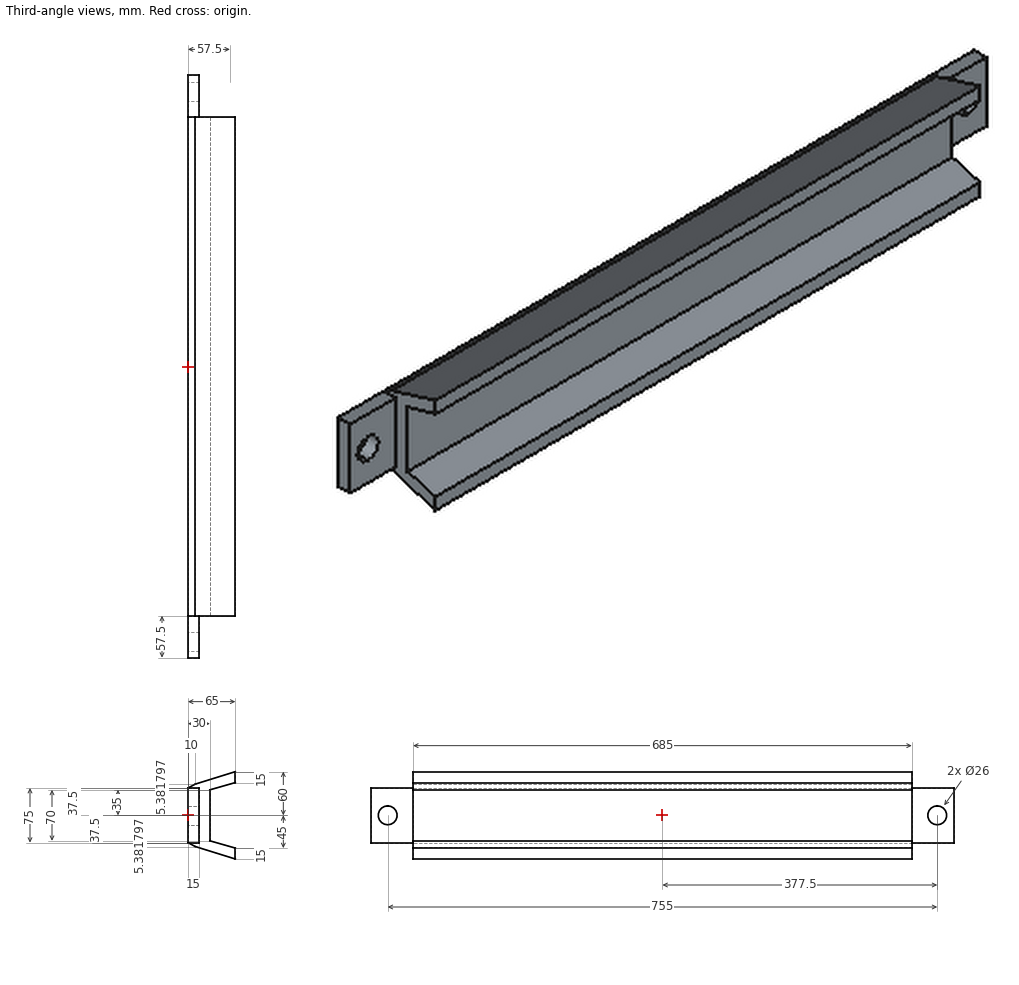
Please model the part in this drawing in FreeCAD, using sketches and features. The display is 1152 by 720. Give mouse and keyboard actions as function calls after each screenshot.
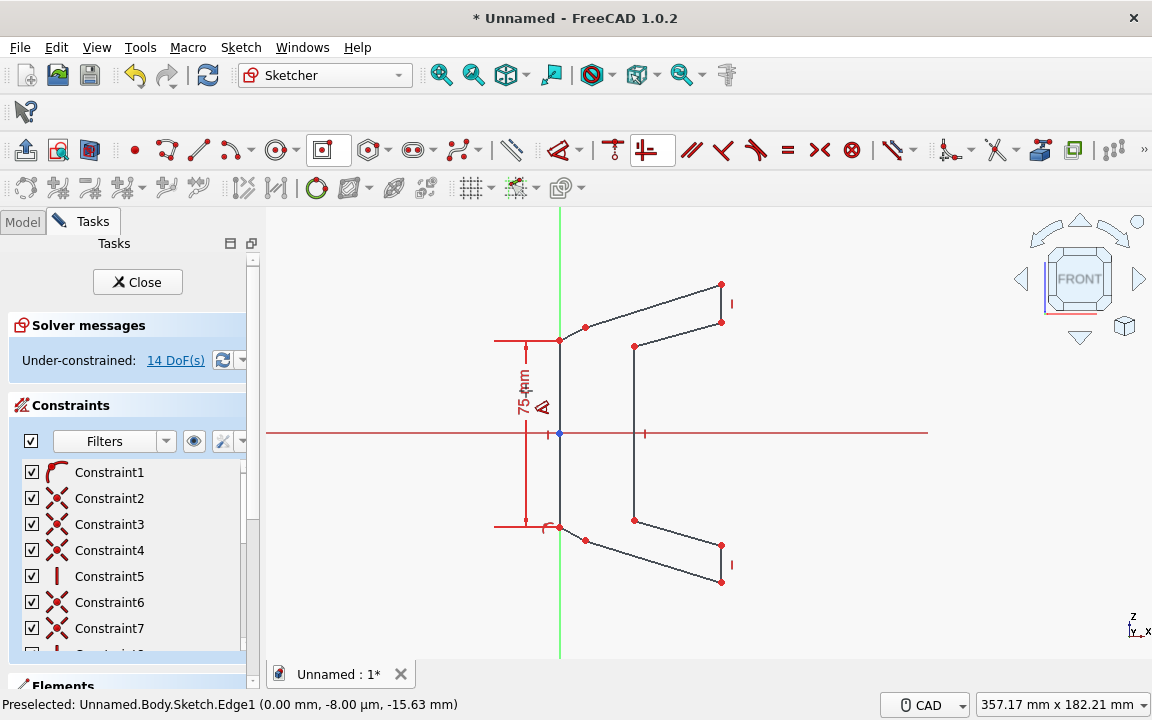
scroll(721, 296, up, 2)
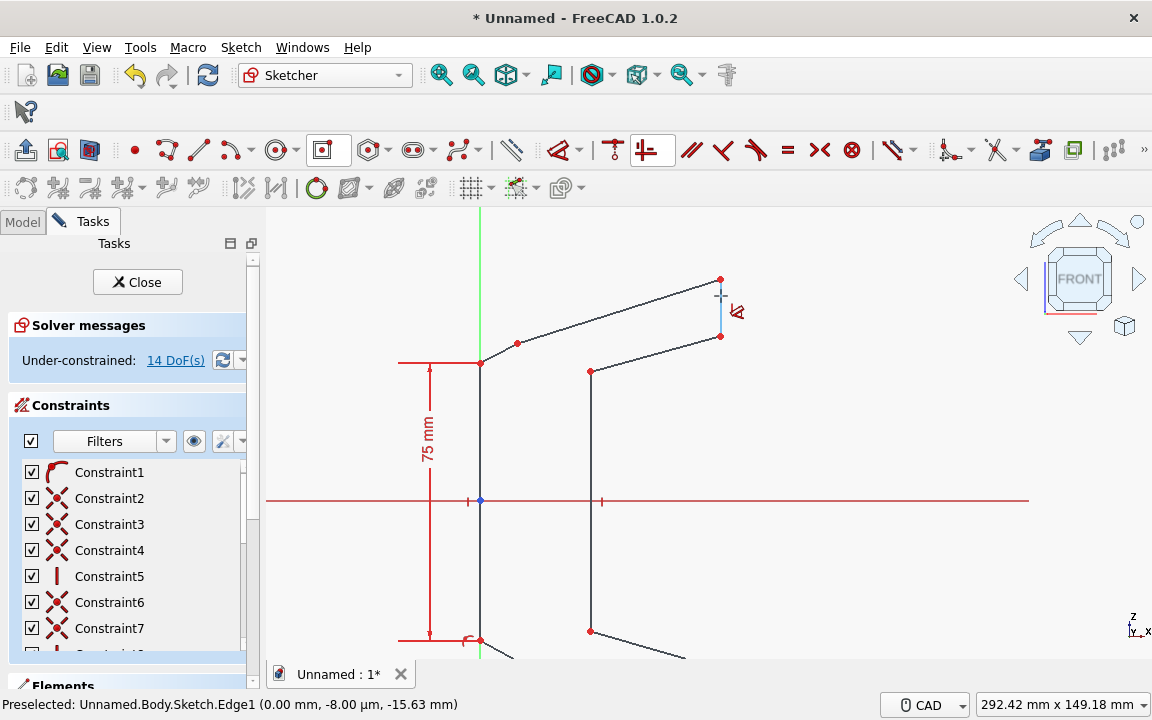
click(721, 296)
click(755, 308)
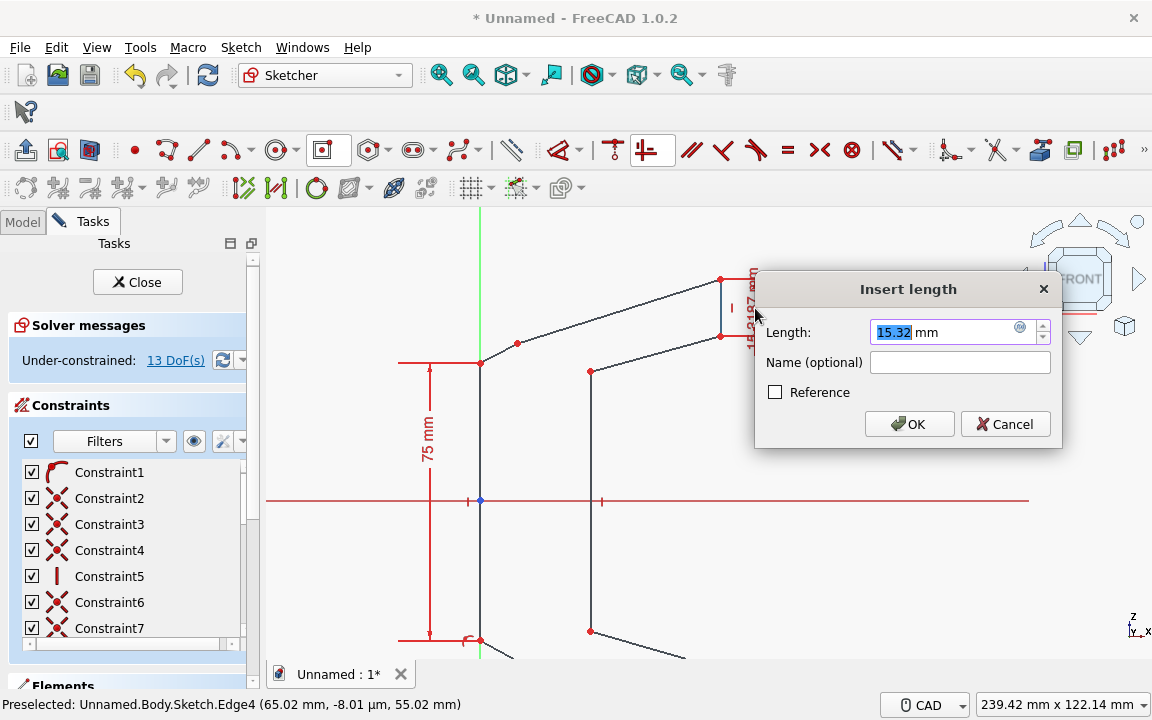
text(15)
key(Return)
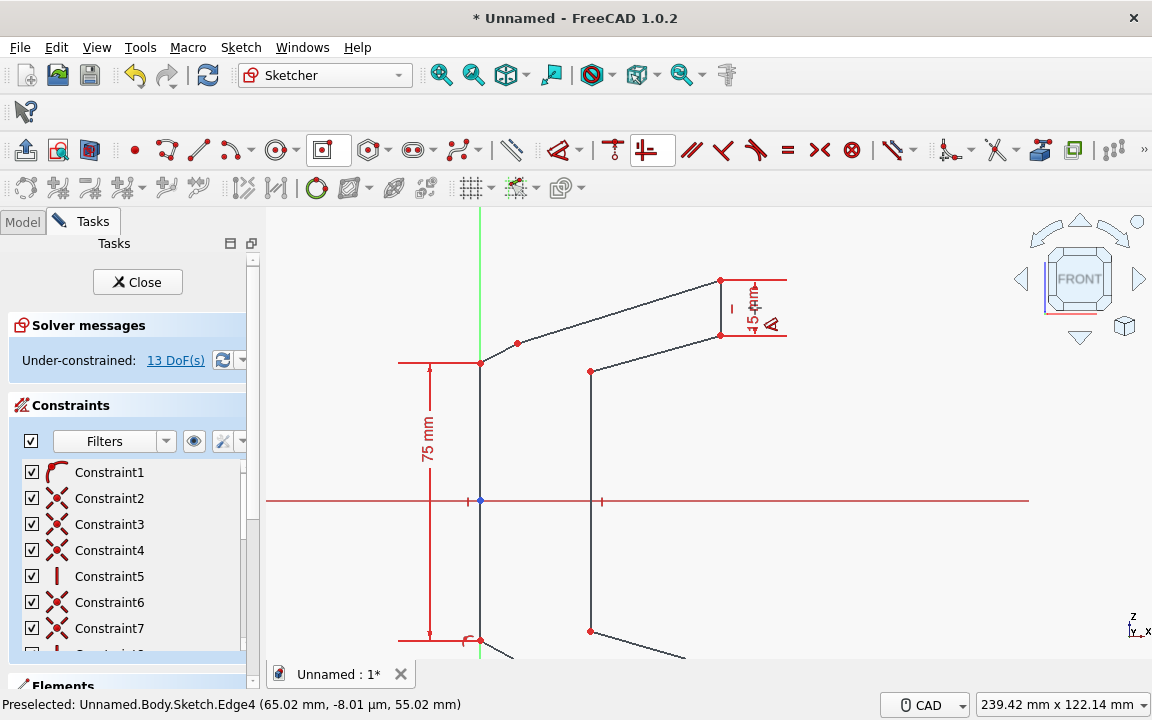
click(591, 450)
click(557, 442)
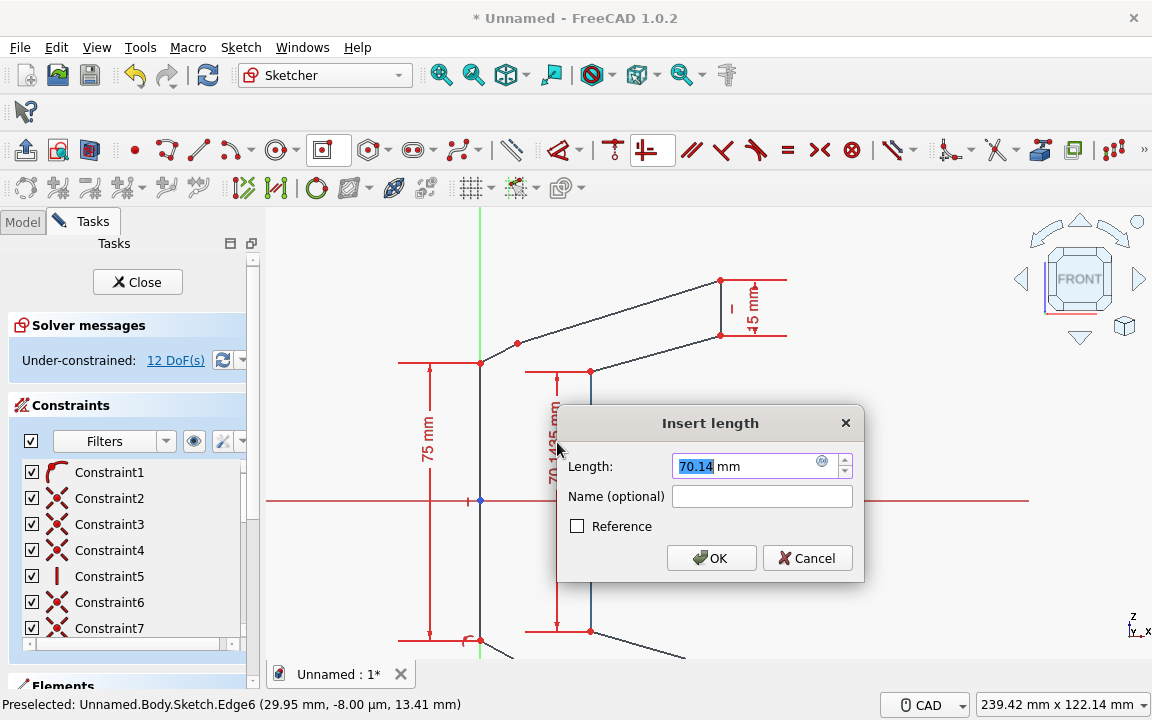
text(70)
key(Return)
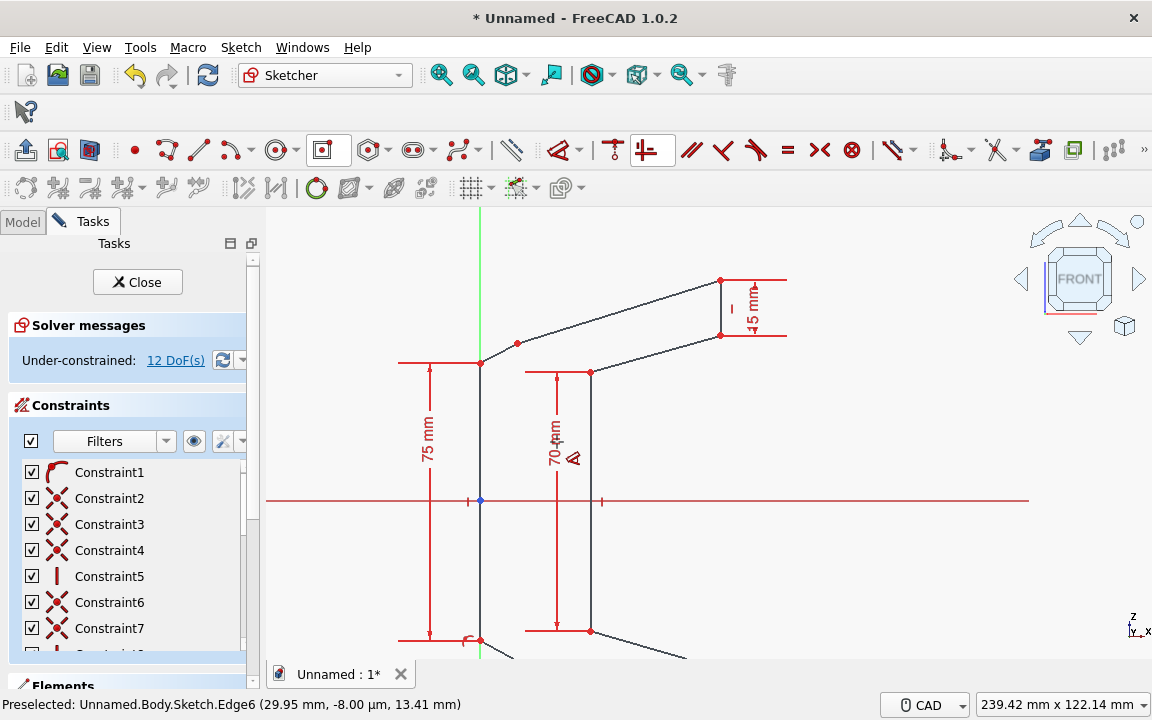
scroll(722, 296, down, 2)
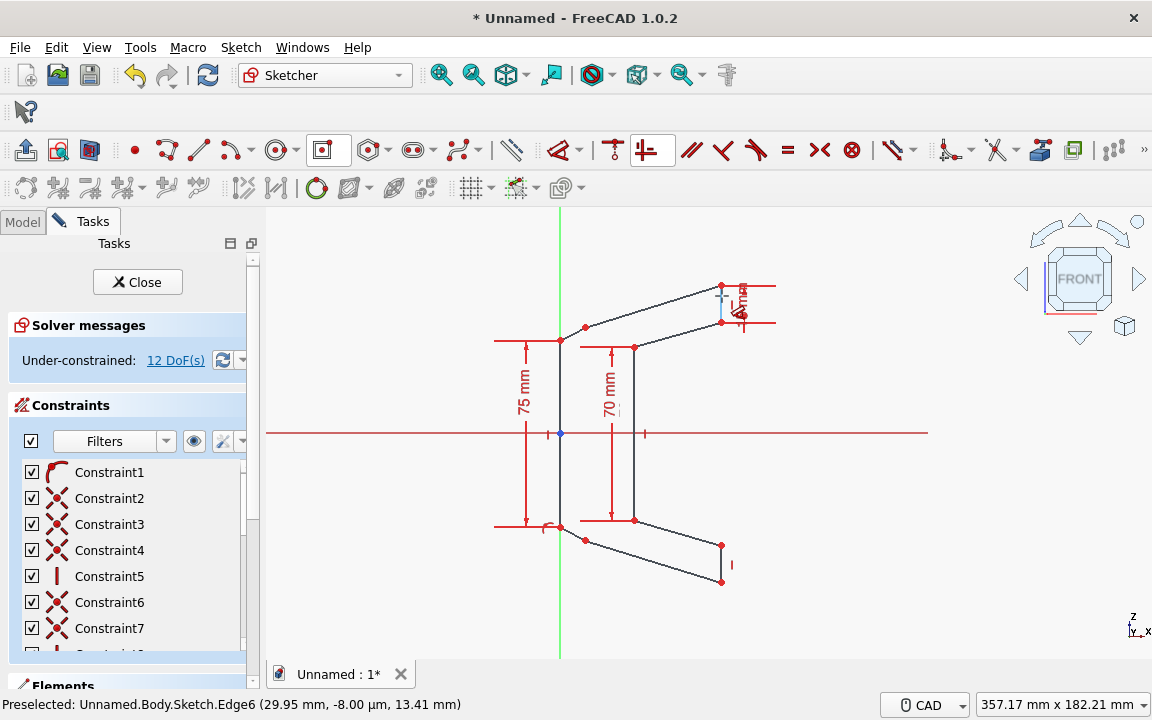
scroll(721, 557, up, 2)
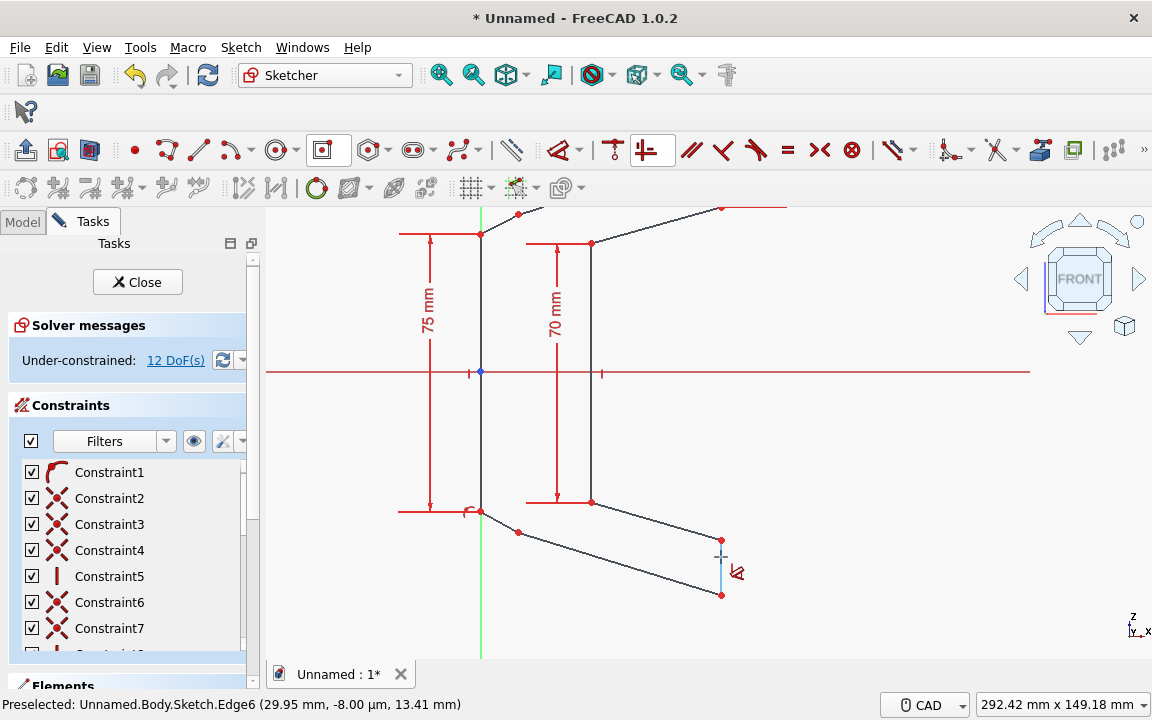
click(721, 557)
click(755, 568)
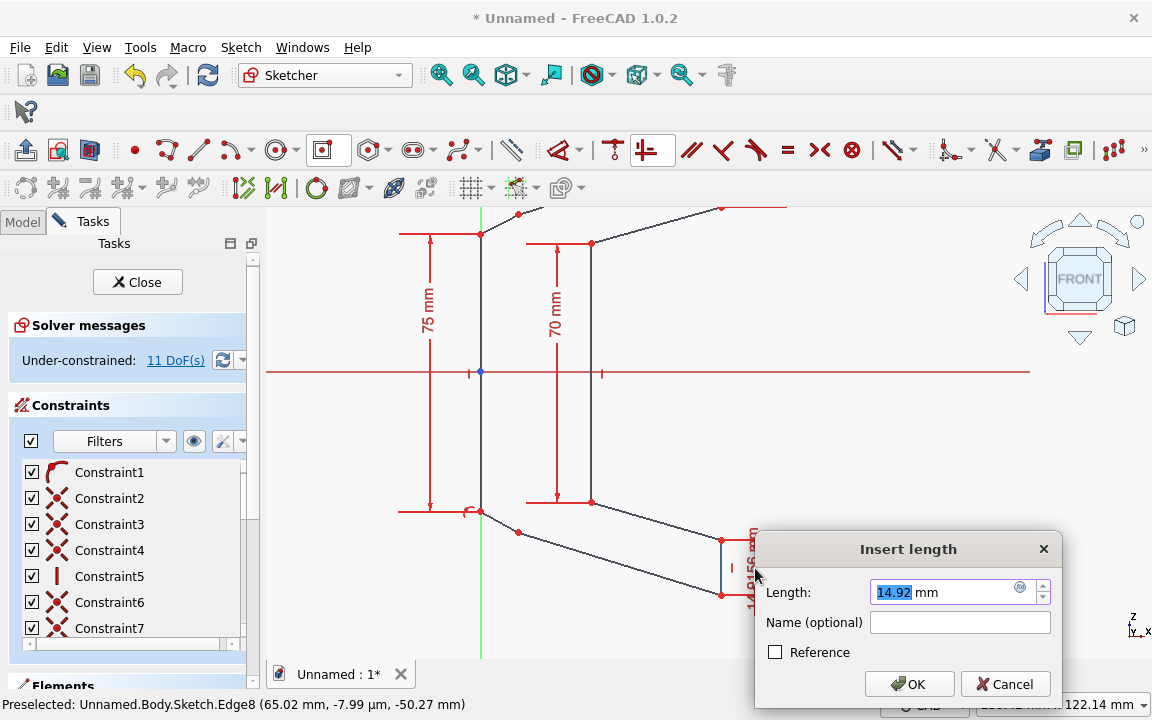
text(15)
key(Return)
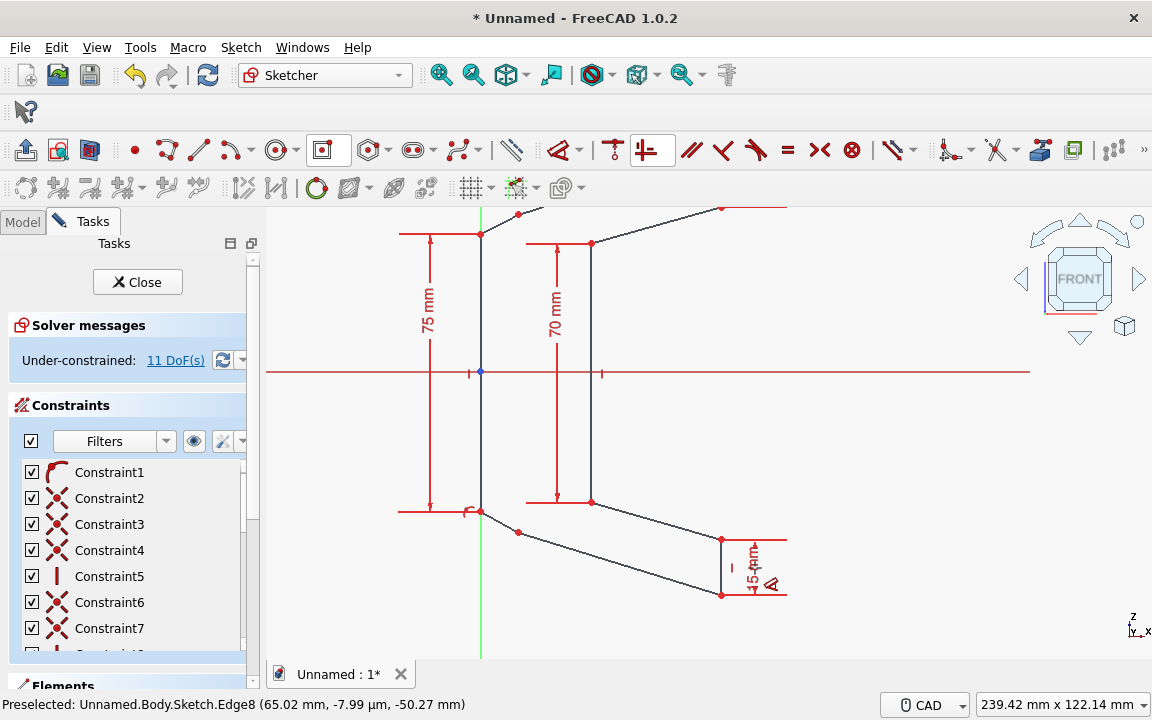
scroll(721, 557, down, 2)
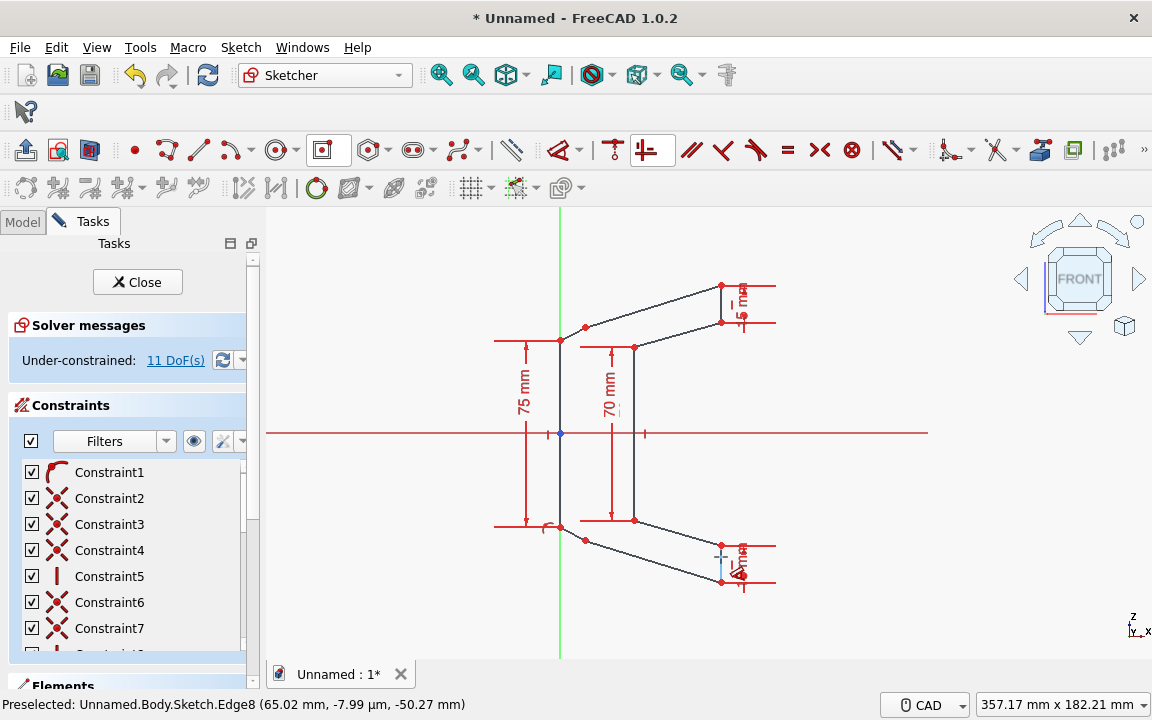
scroll(585, 328, up, 3)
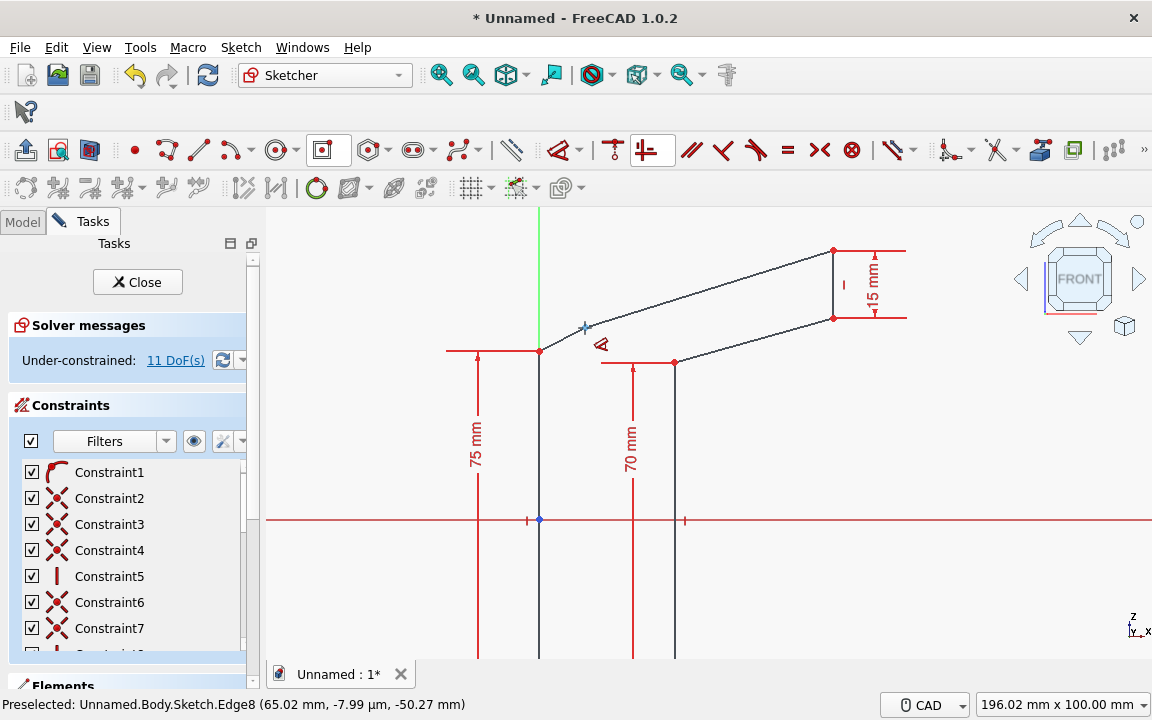
click(585, 328)
click(562, 294)